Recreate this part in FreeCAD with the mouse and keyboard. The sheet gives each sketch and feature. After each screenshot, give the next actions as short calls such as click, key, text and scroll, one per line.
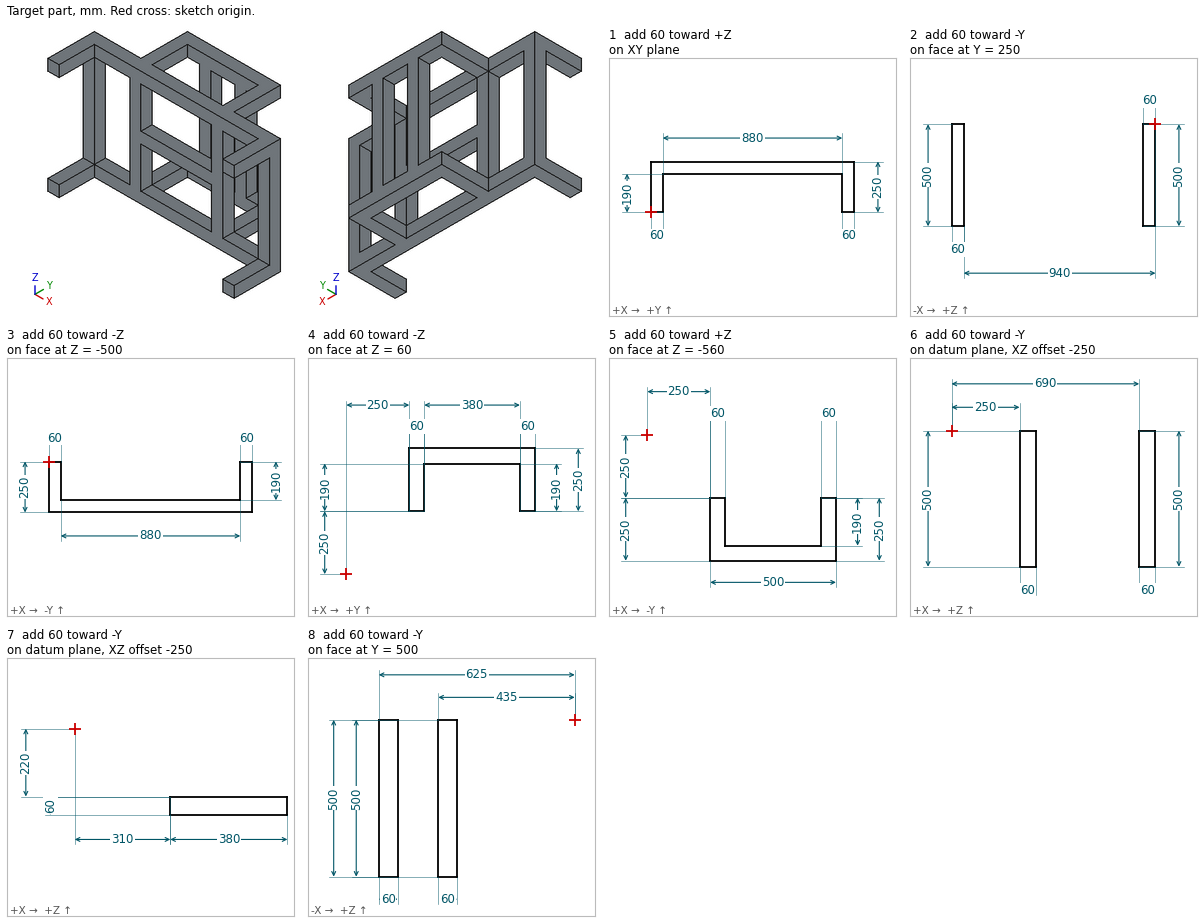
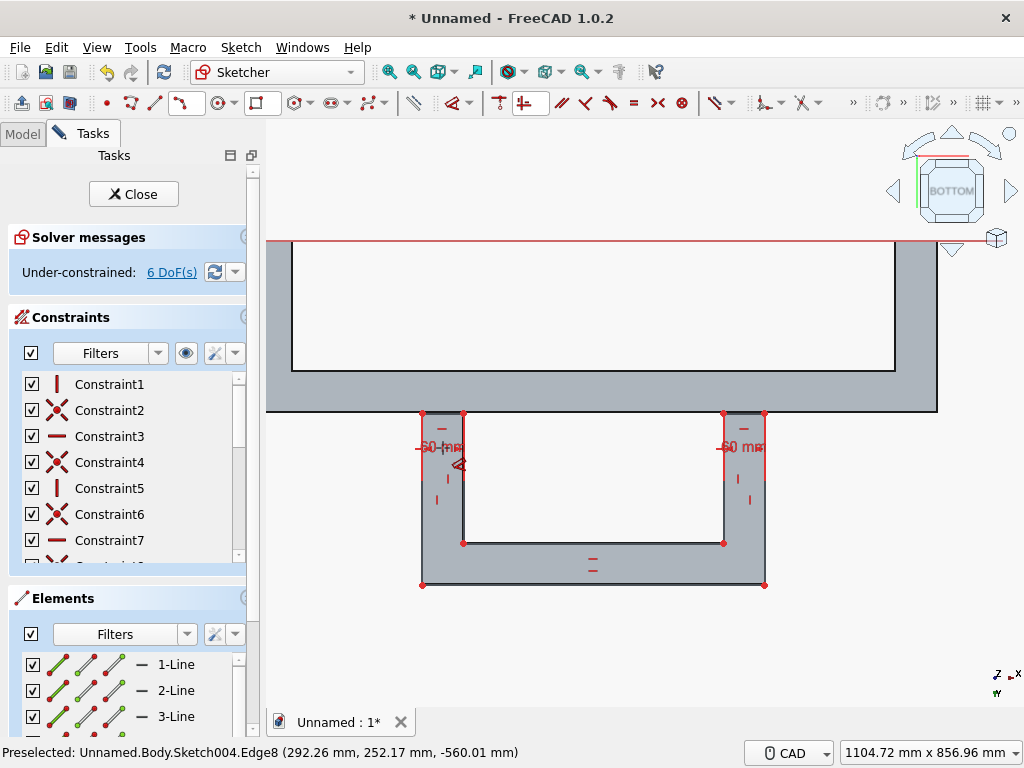
click(422, 465)
click(388, 500)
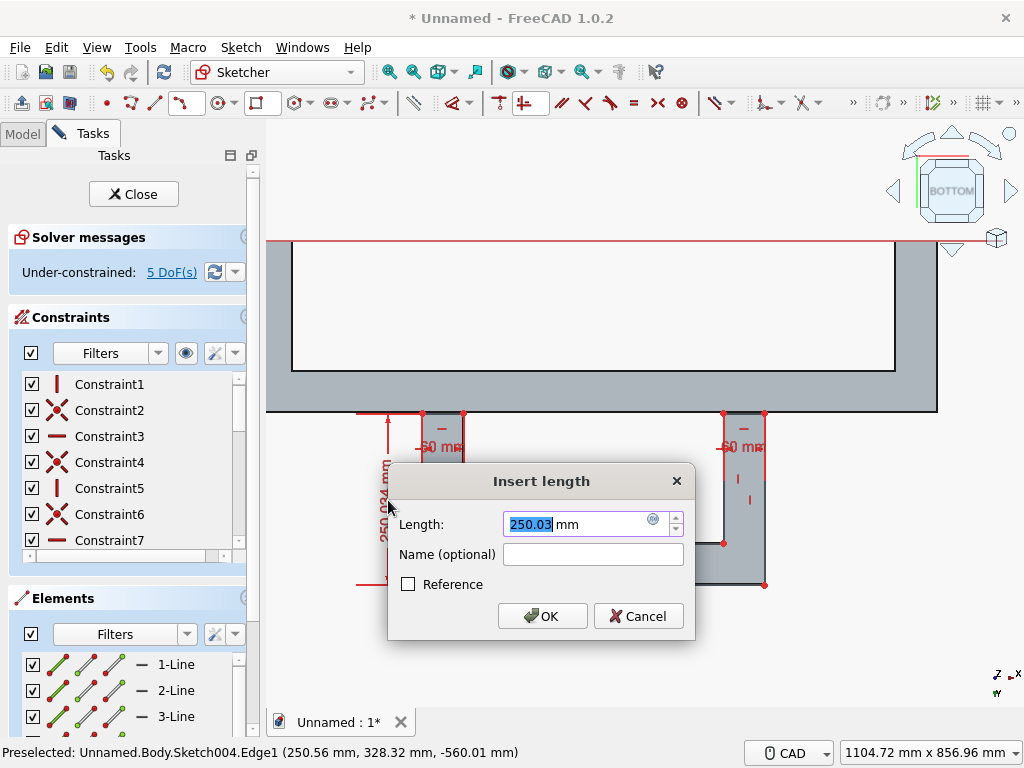
text(250)
key(Return)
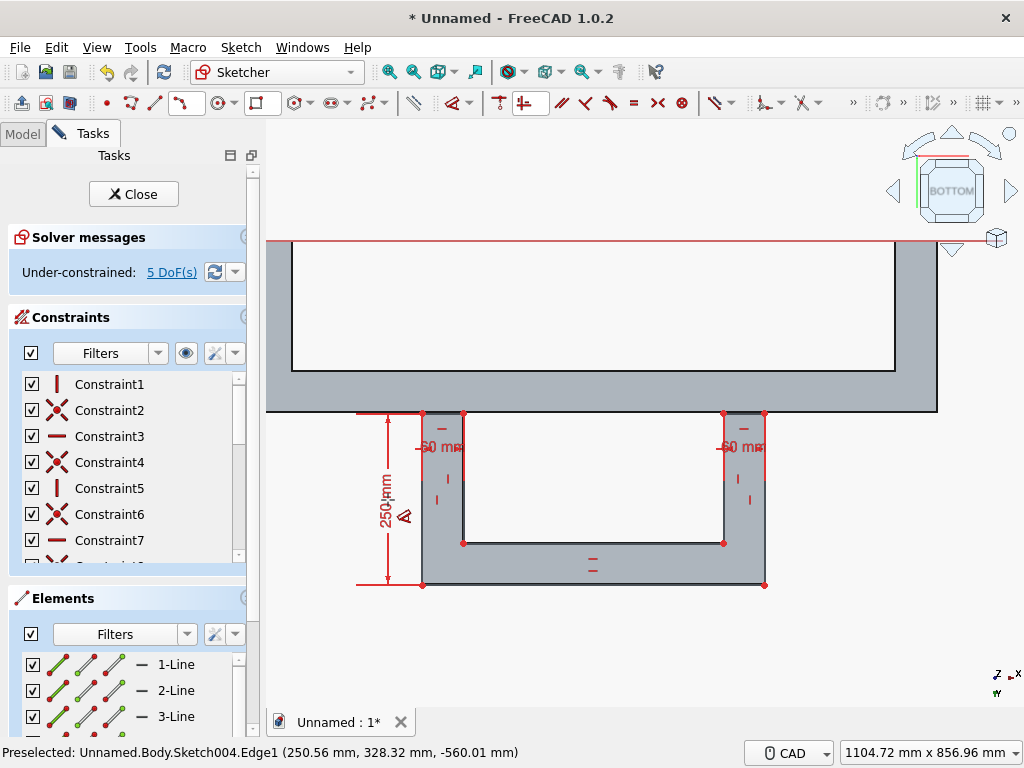
click(525, 585)
click(594, 619)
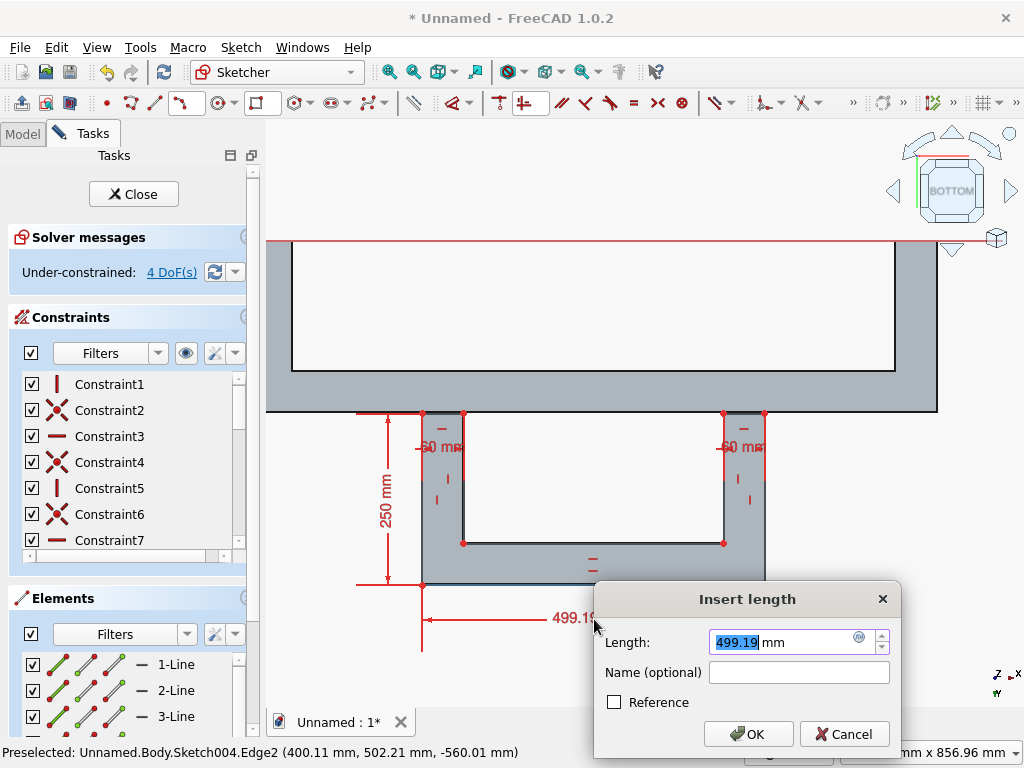
text(500)
key(Return)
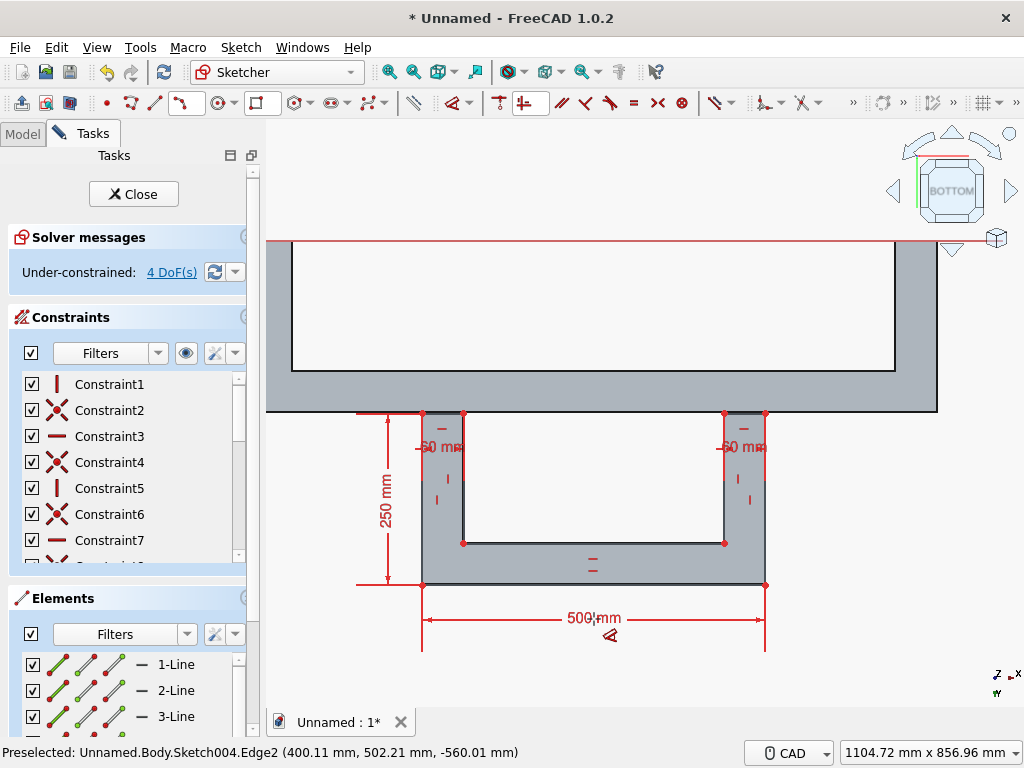
click(765, 534)
click(799, 500)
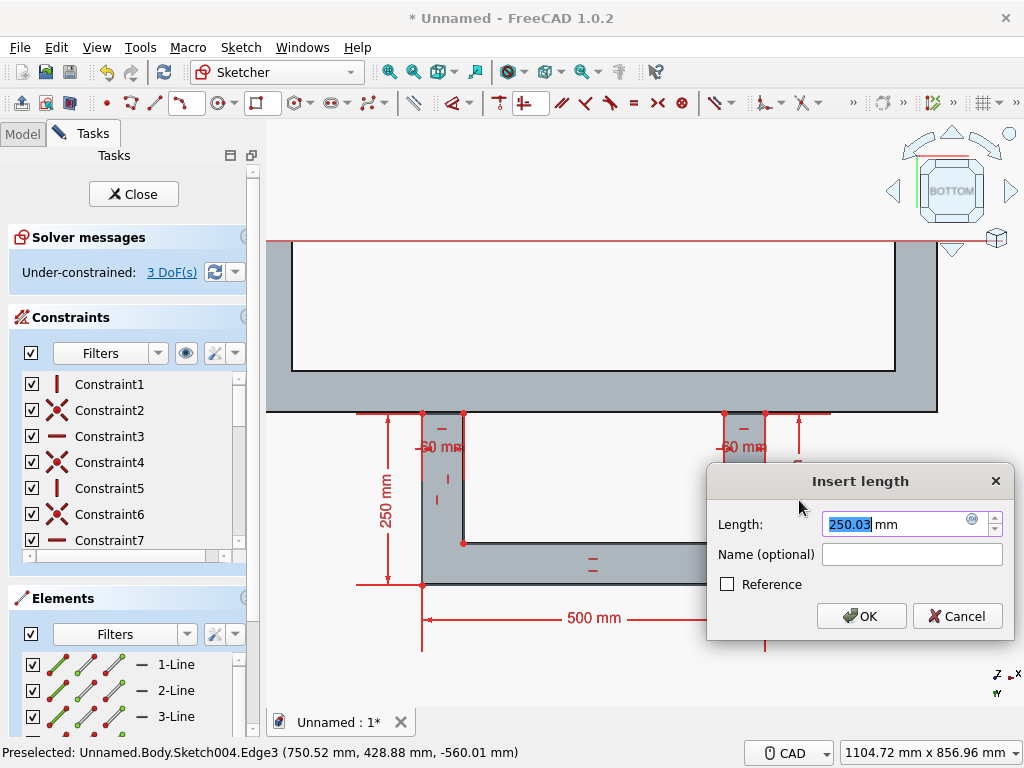
text(250)
key(Return)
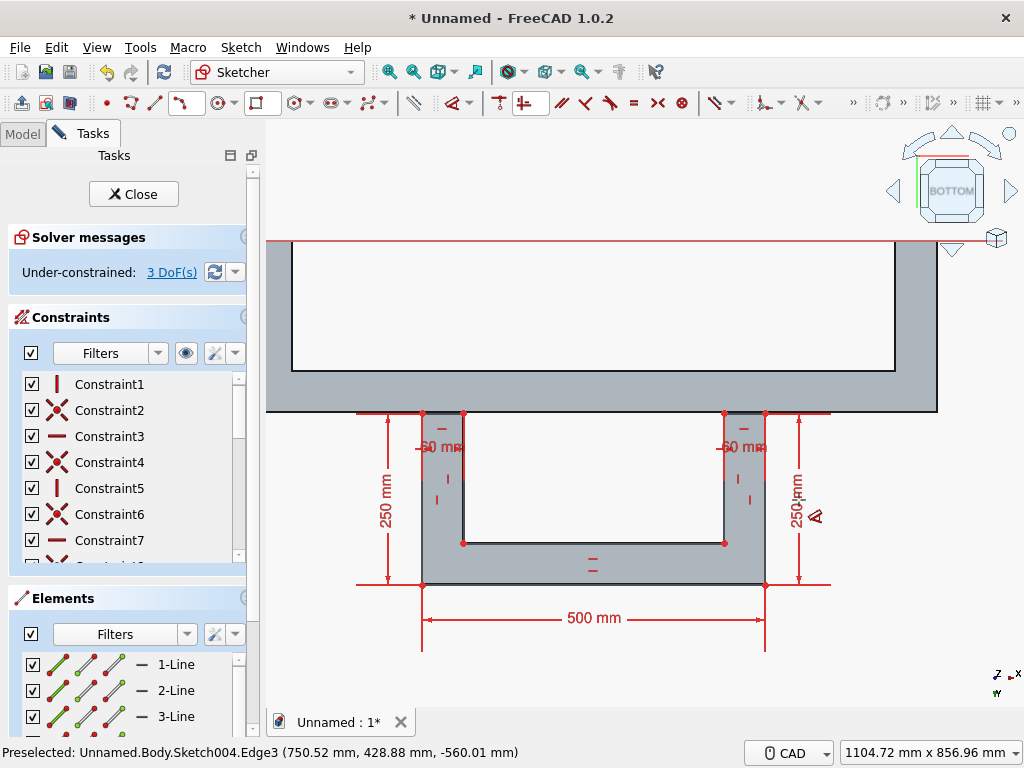
click(724, 453)
click(690, 479)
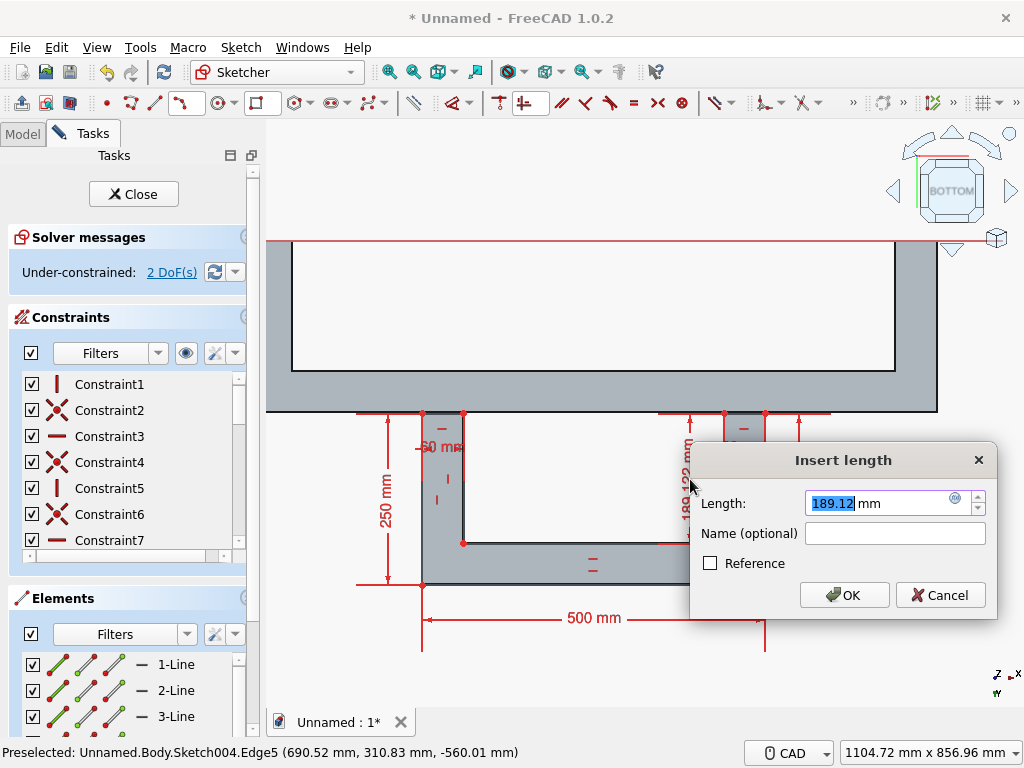
text(190)
key(Return)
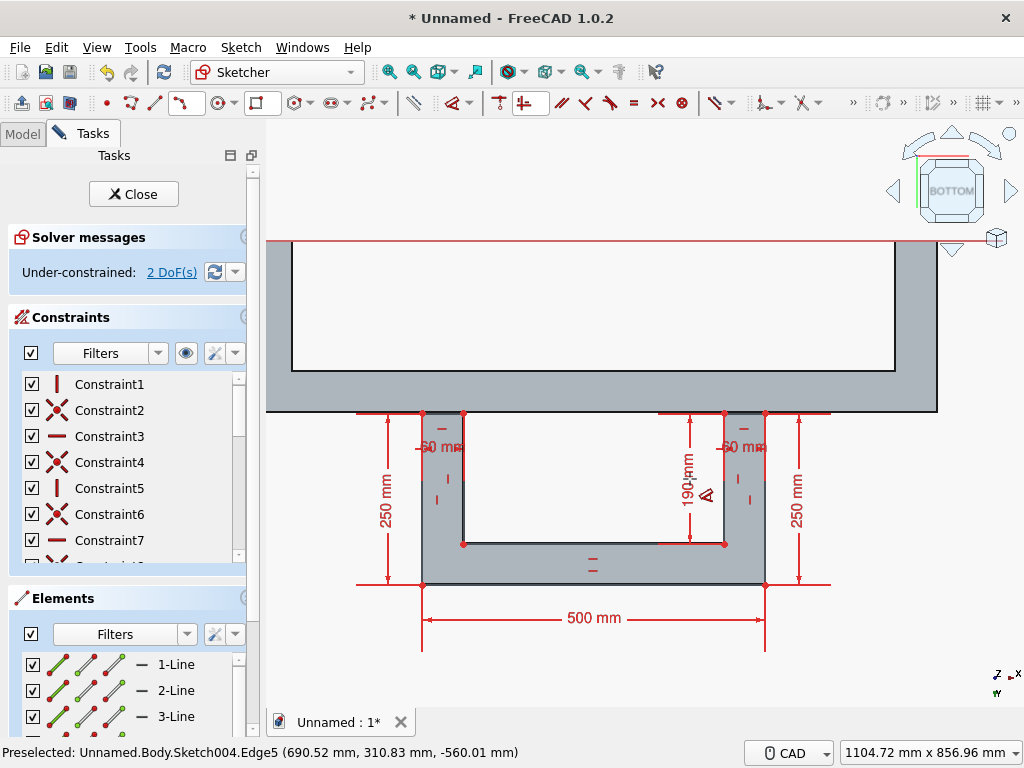
click(422, 414)
click(358, 207)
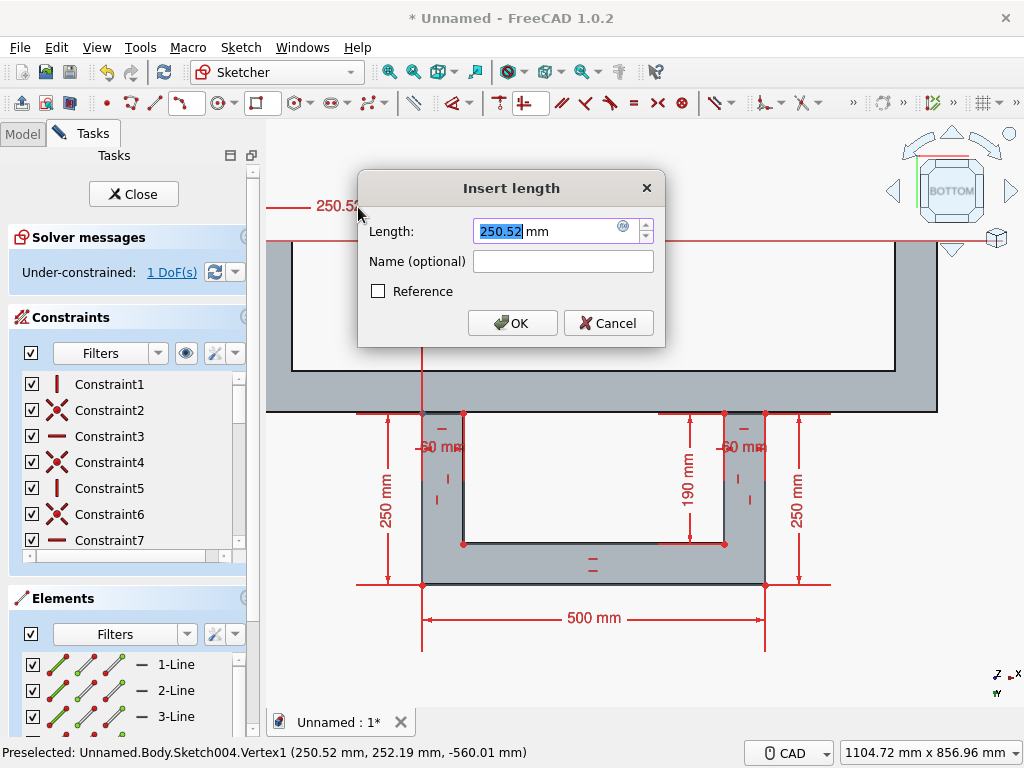
text(250)
key(Return)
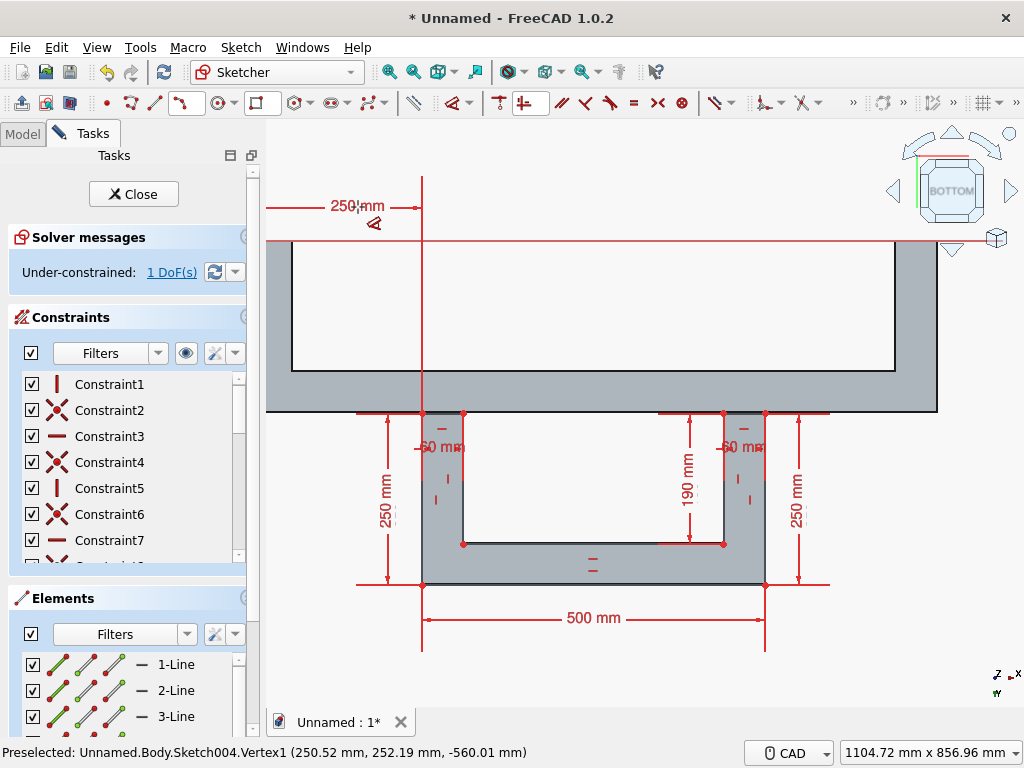
click(422, 414)
click(456, 327)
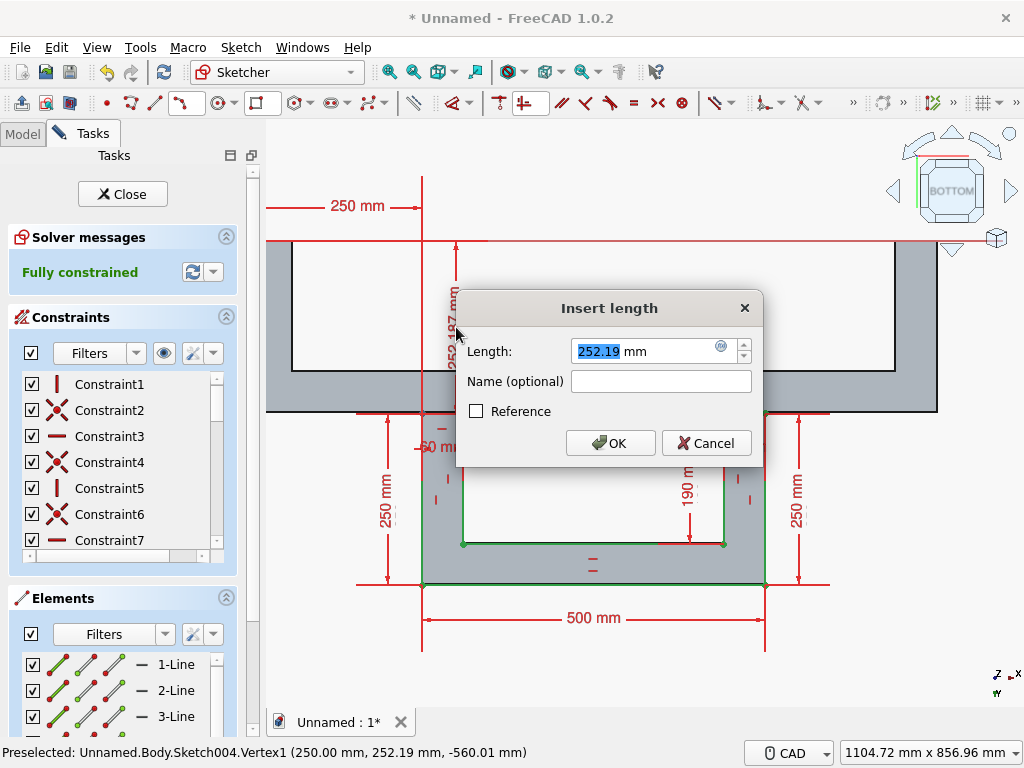
text(250)
key(Return)
key(Escape)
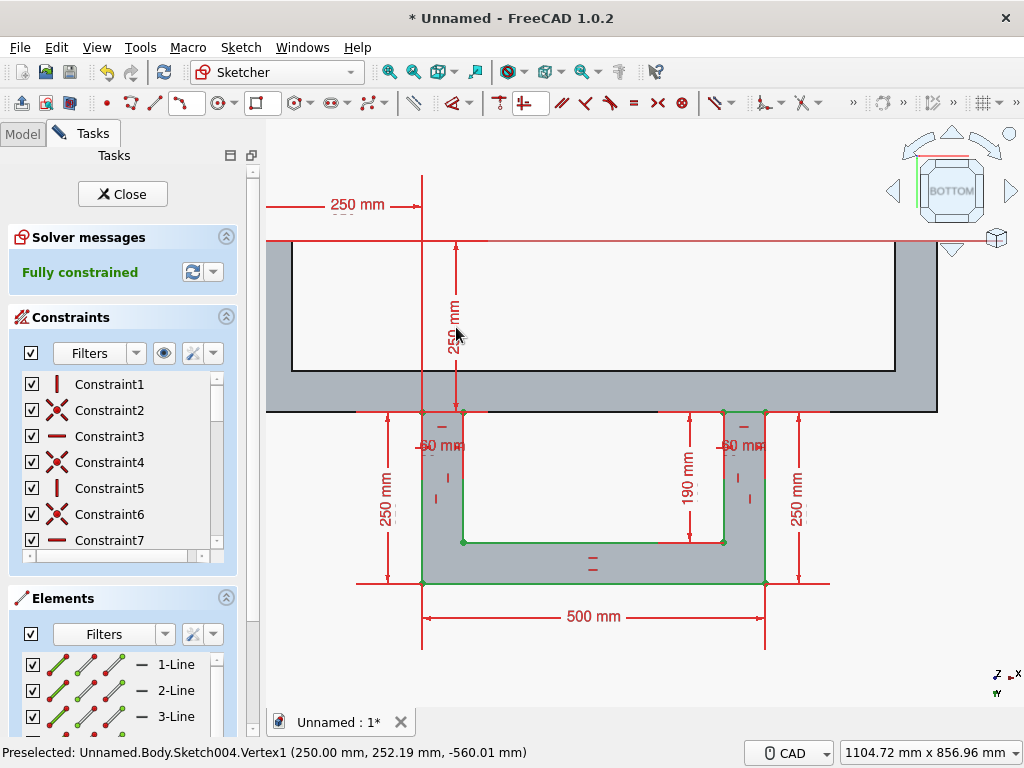
click(123, 194)